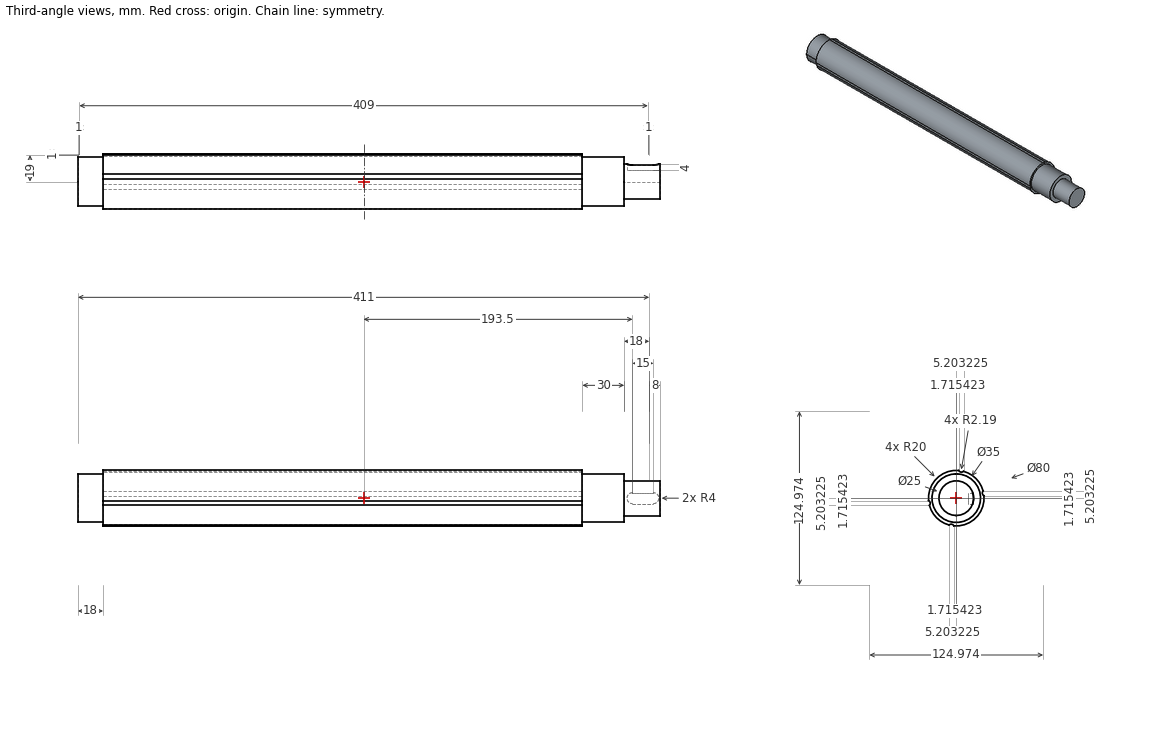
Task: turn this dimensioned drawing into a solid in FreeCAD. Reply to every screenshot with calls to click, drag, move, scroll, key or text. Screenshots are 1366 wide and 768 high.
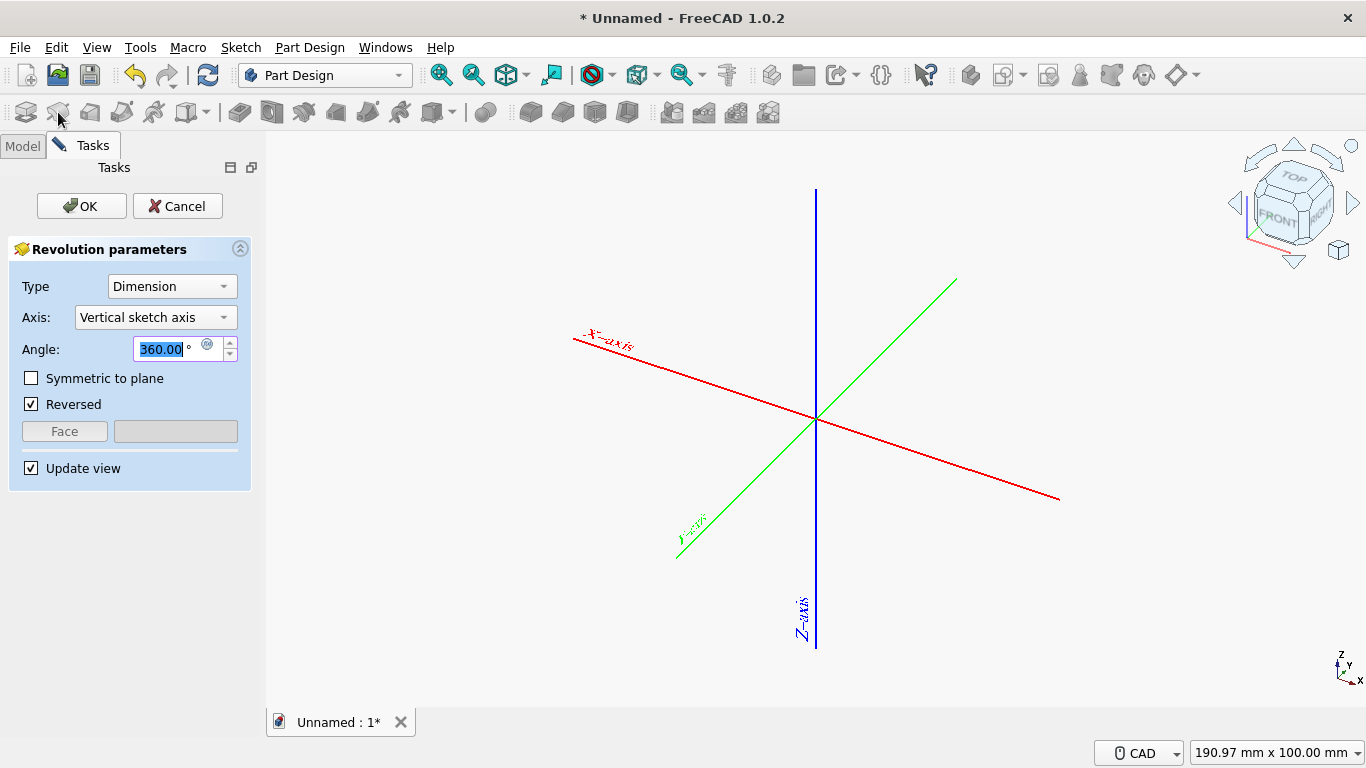
click(156, 318)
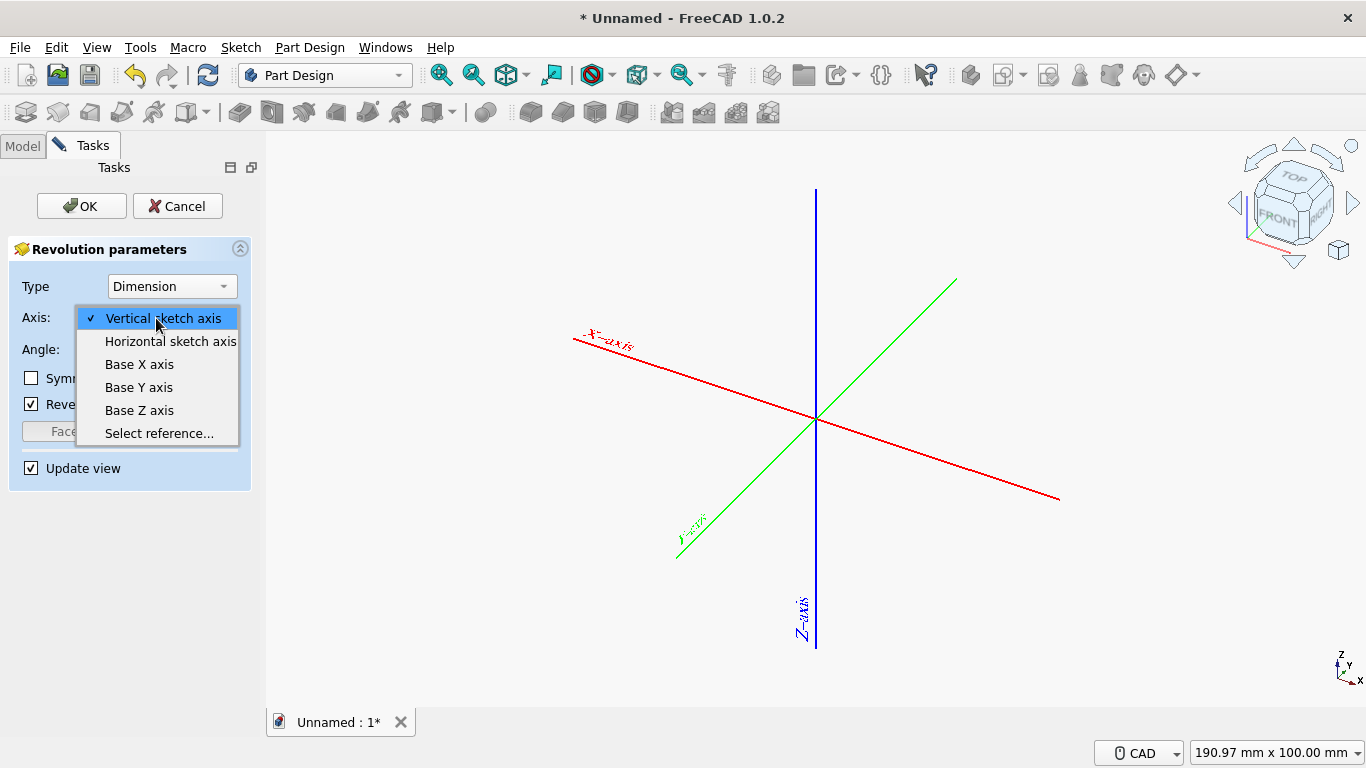
click(156, 342)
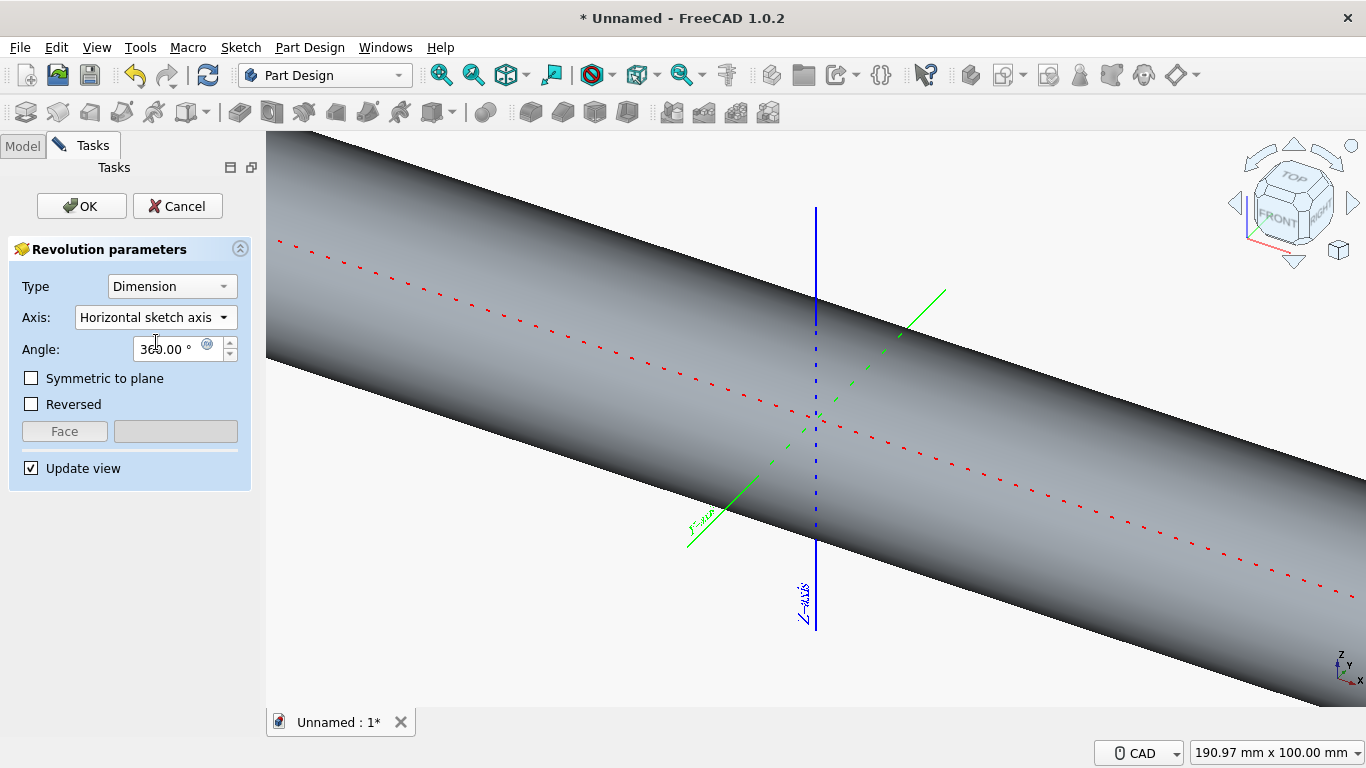
click(82, 206)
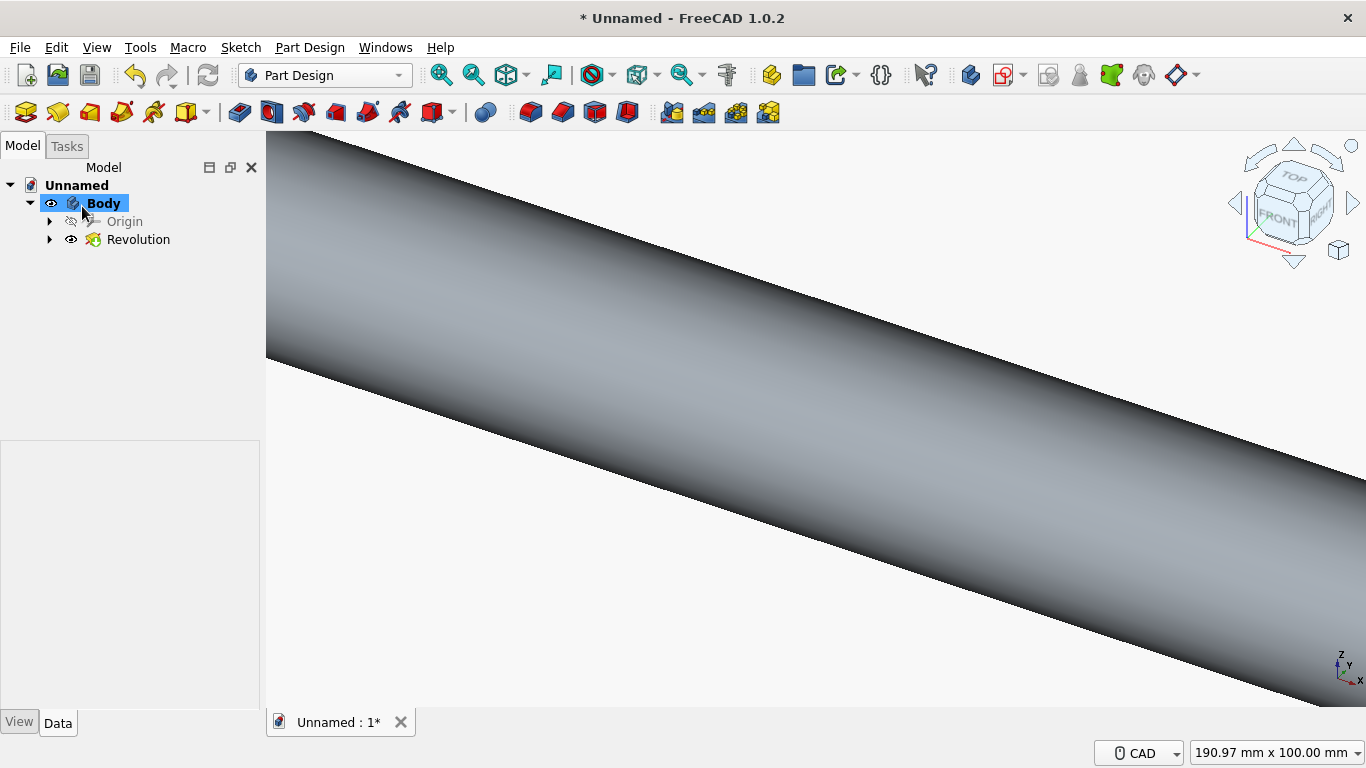
key(v)
key(f)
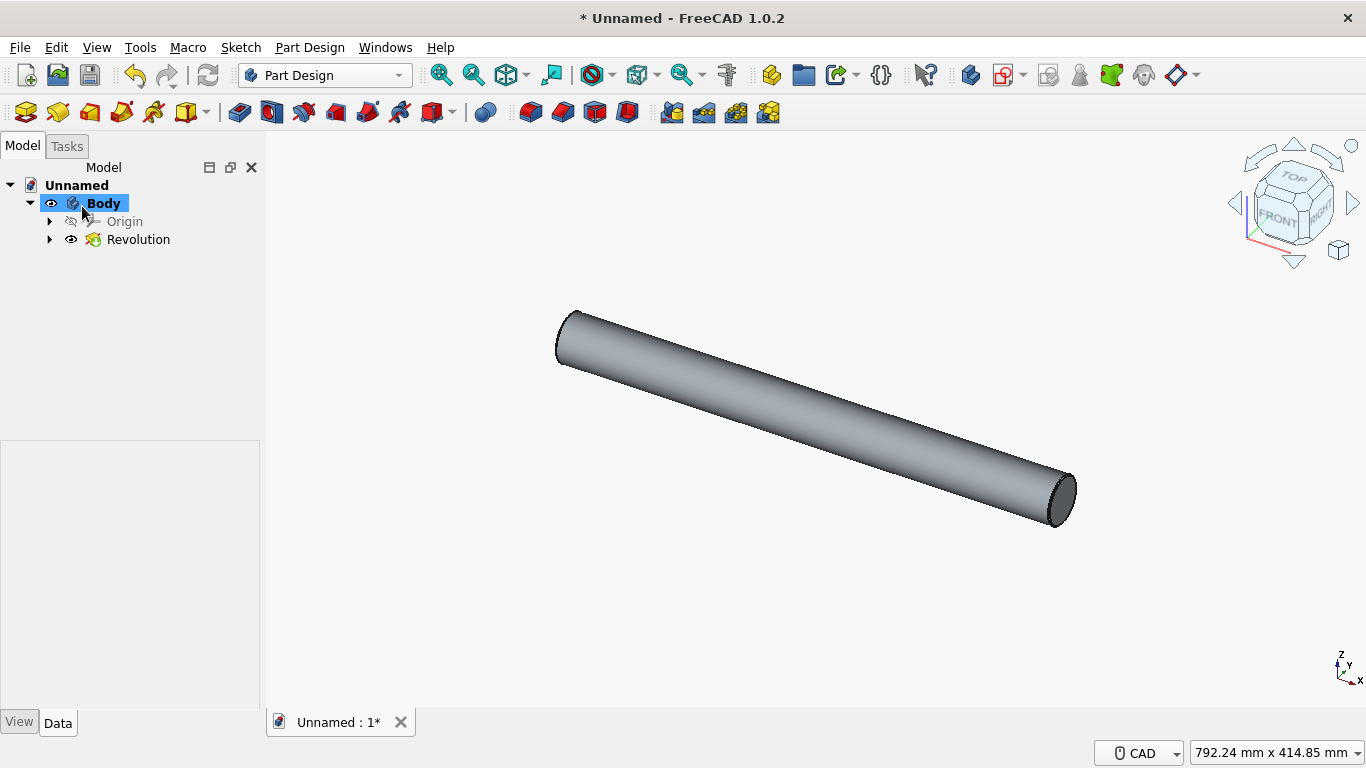
click(1004, 76)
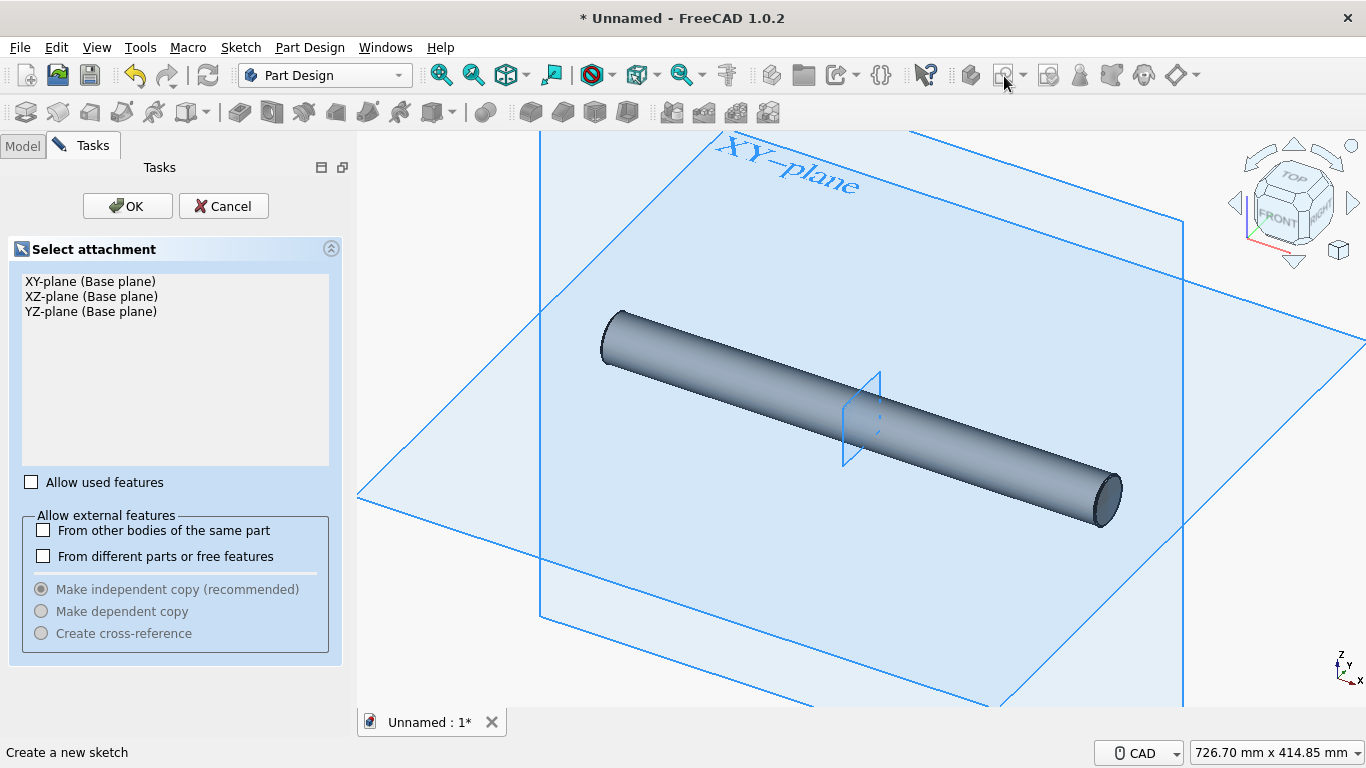
click(82, 312)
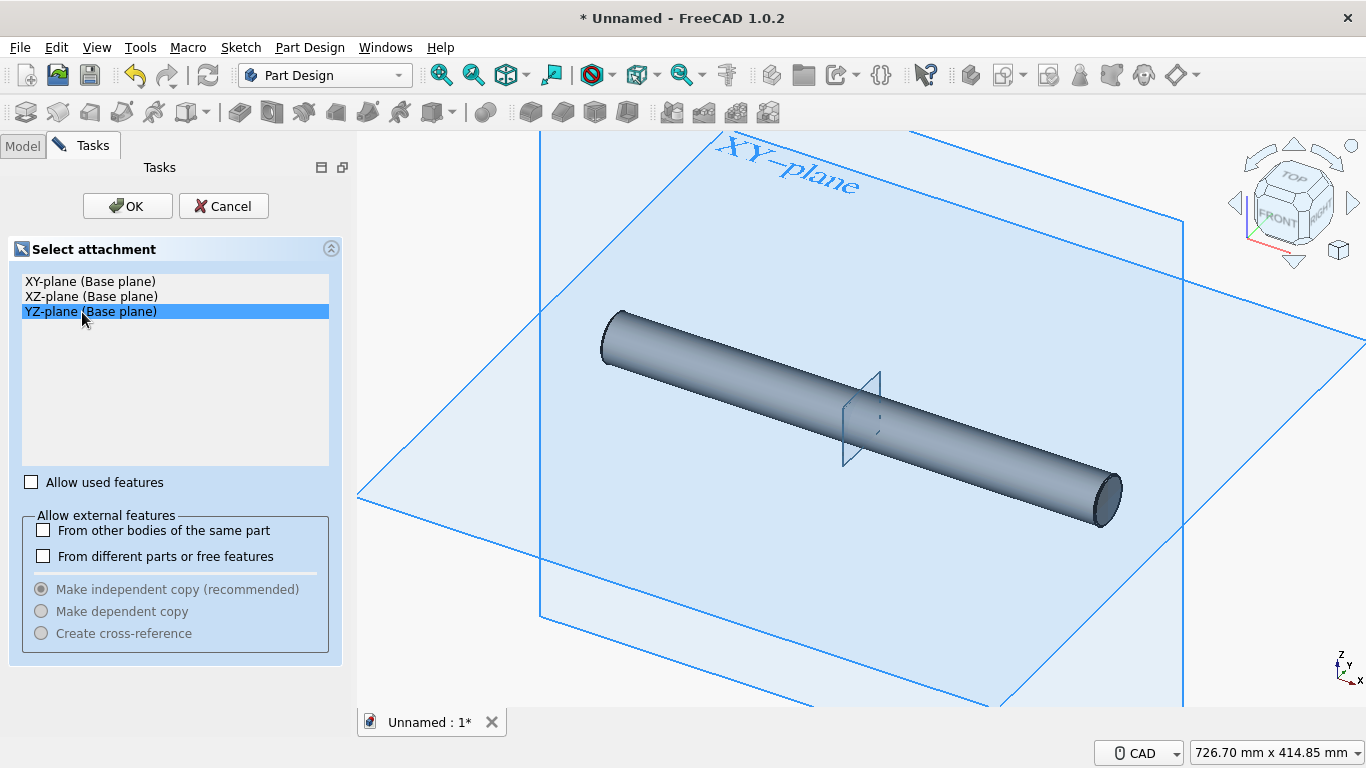
click(128, 206)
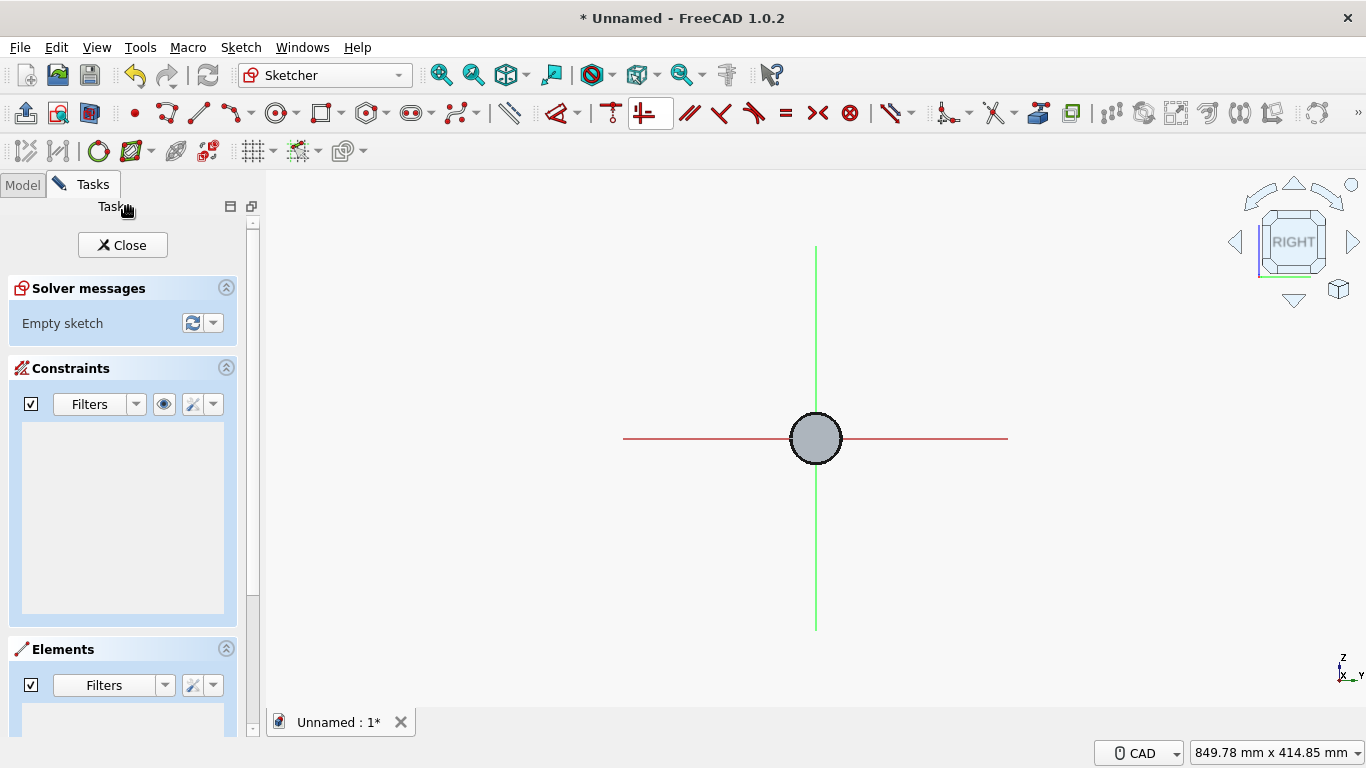
click(90, 114)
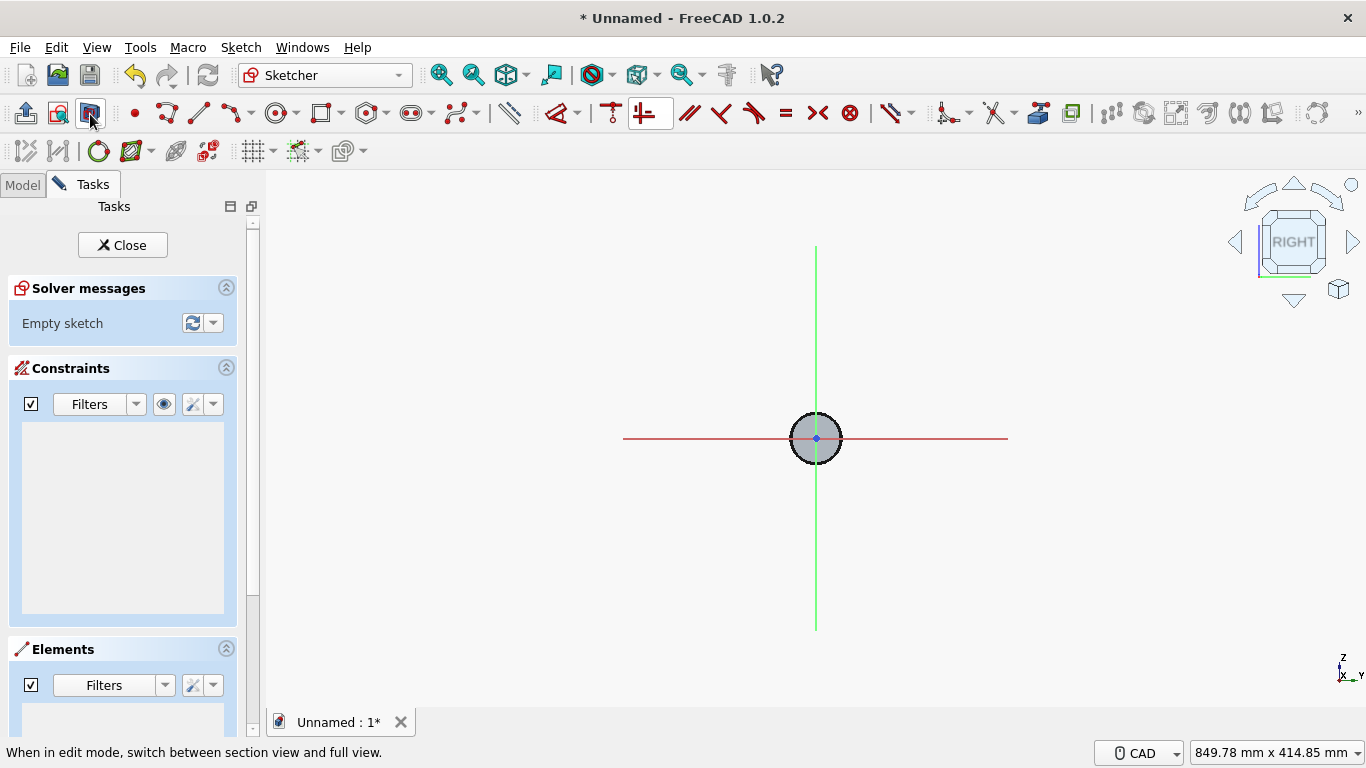
scroll(846, 438, up, 6)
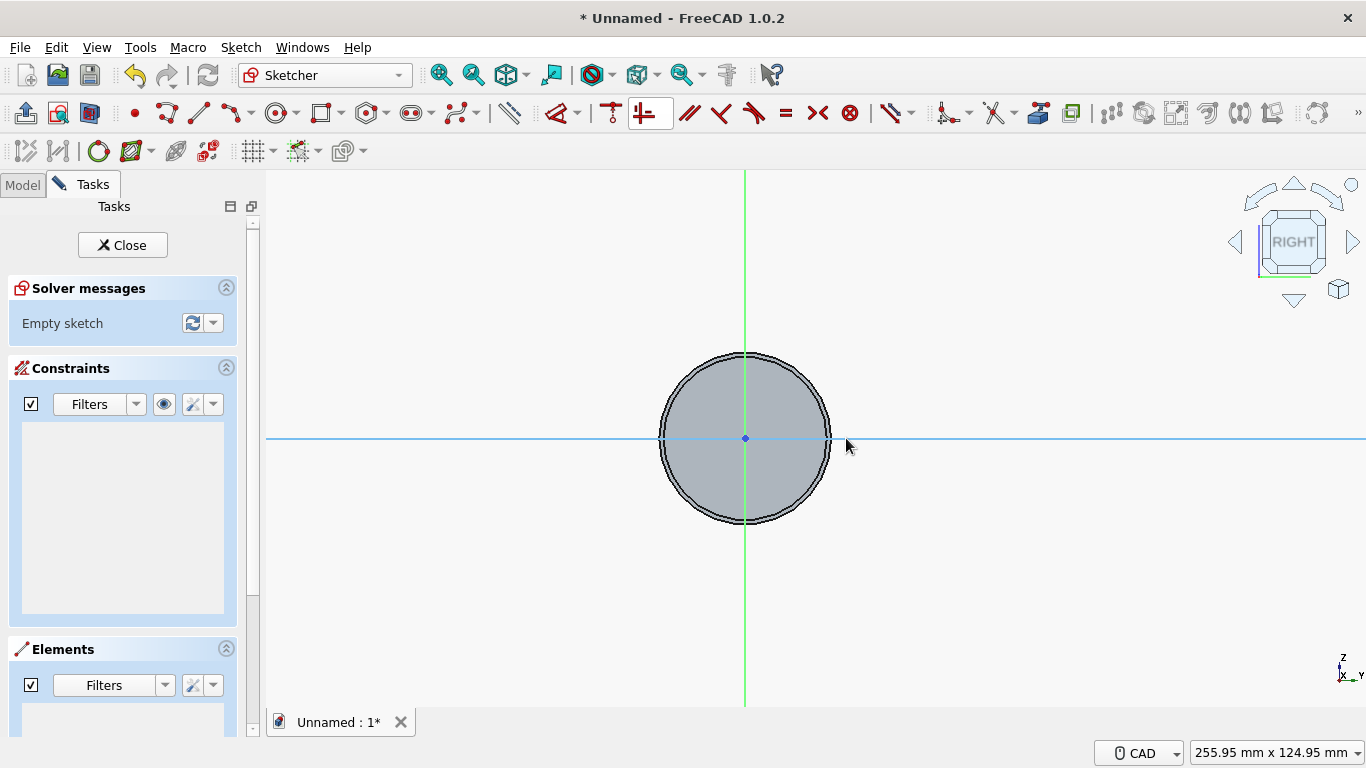
click(232, 114)